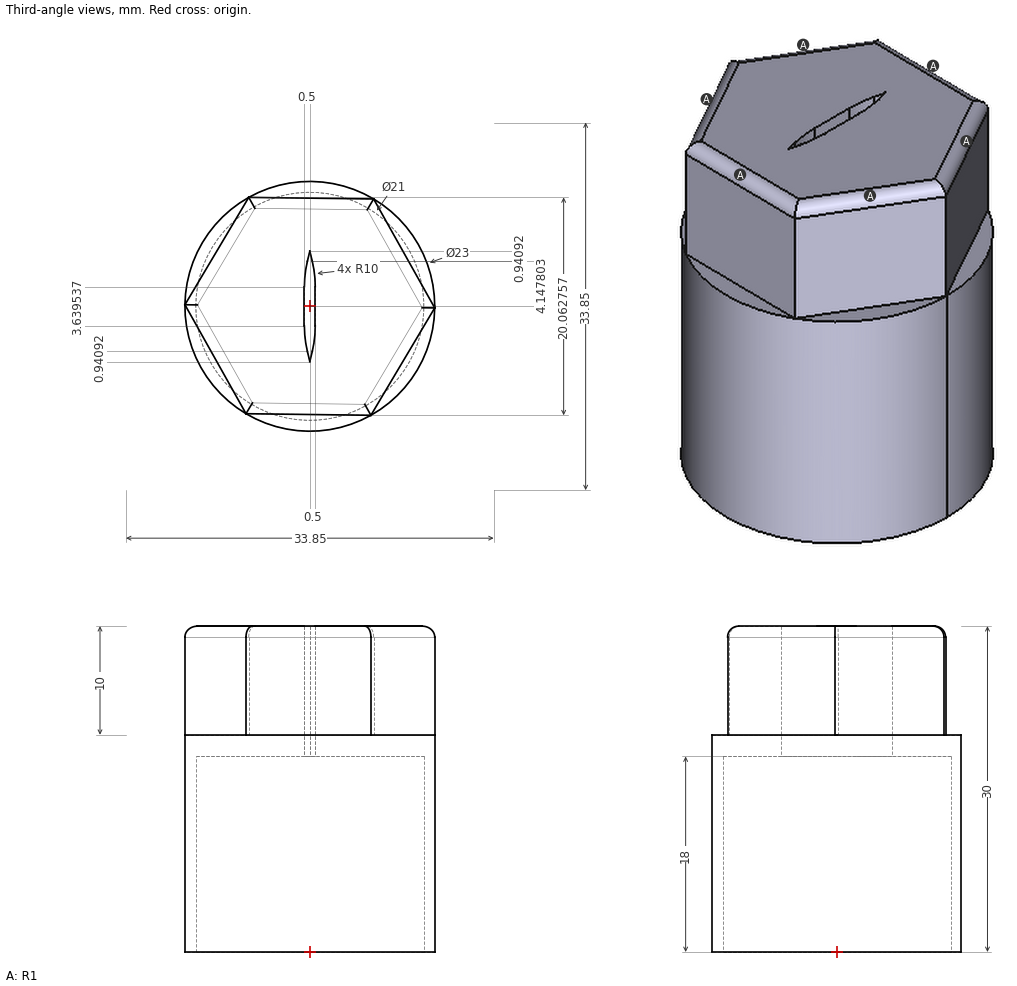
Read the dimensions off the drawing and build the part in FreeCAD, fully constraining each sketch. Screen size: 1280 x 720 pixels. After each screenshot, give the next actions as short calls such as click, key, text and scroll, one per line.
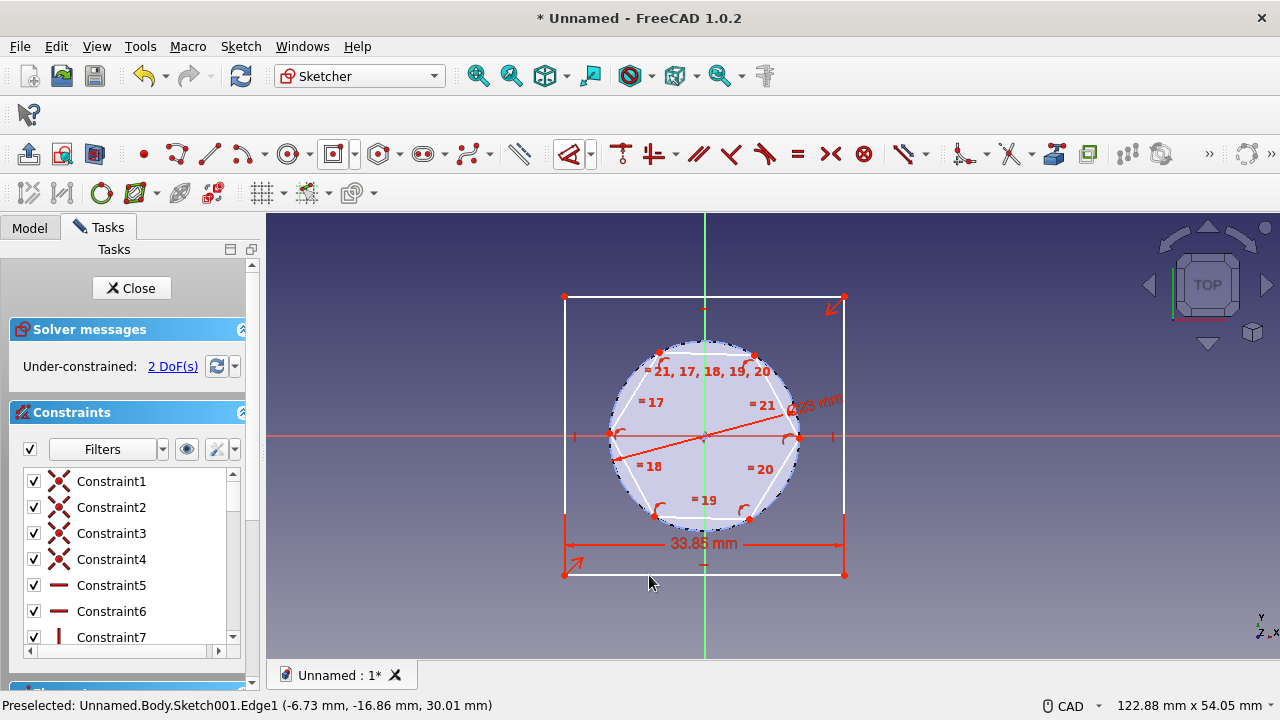
click(844, 492)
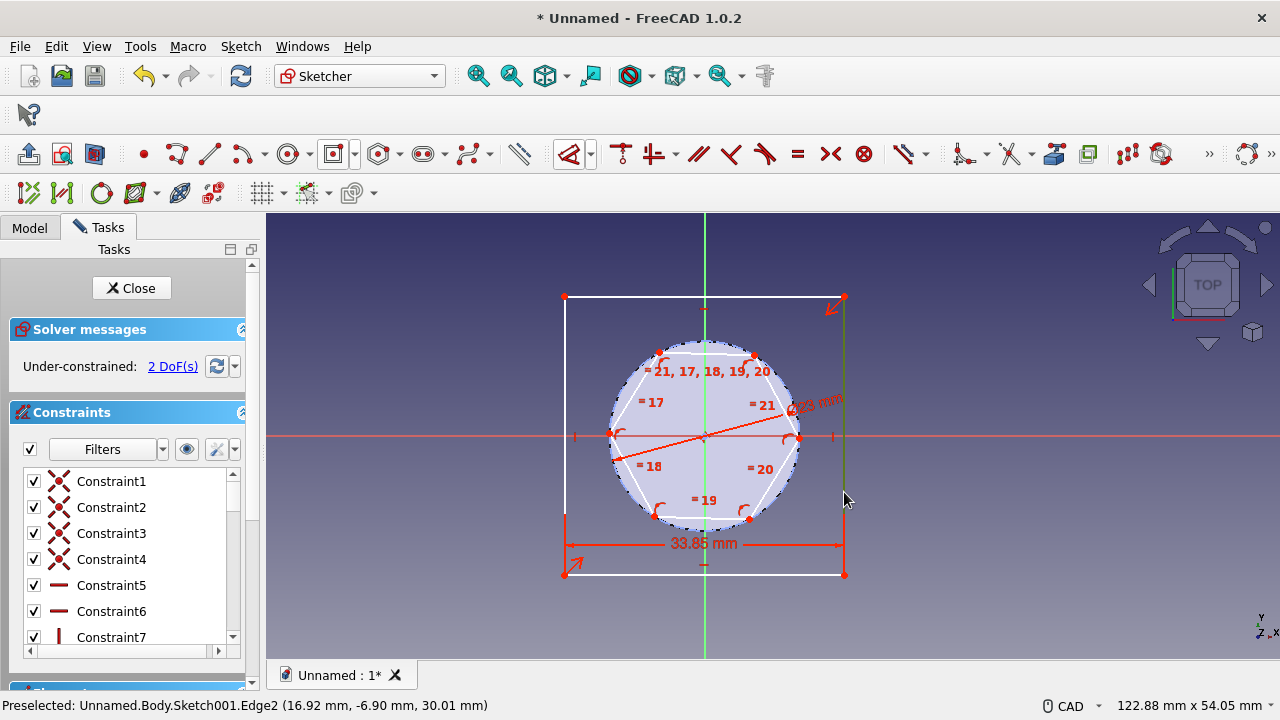
key(i)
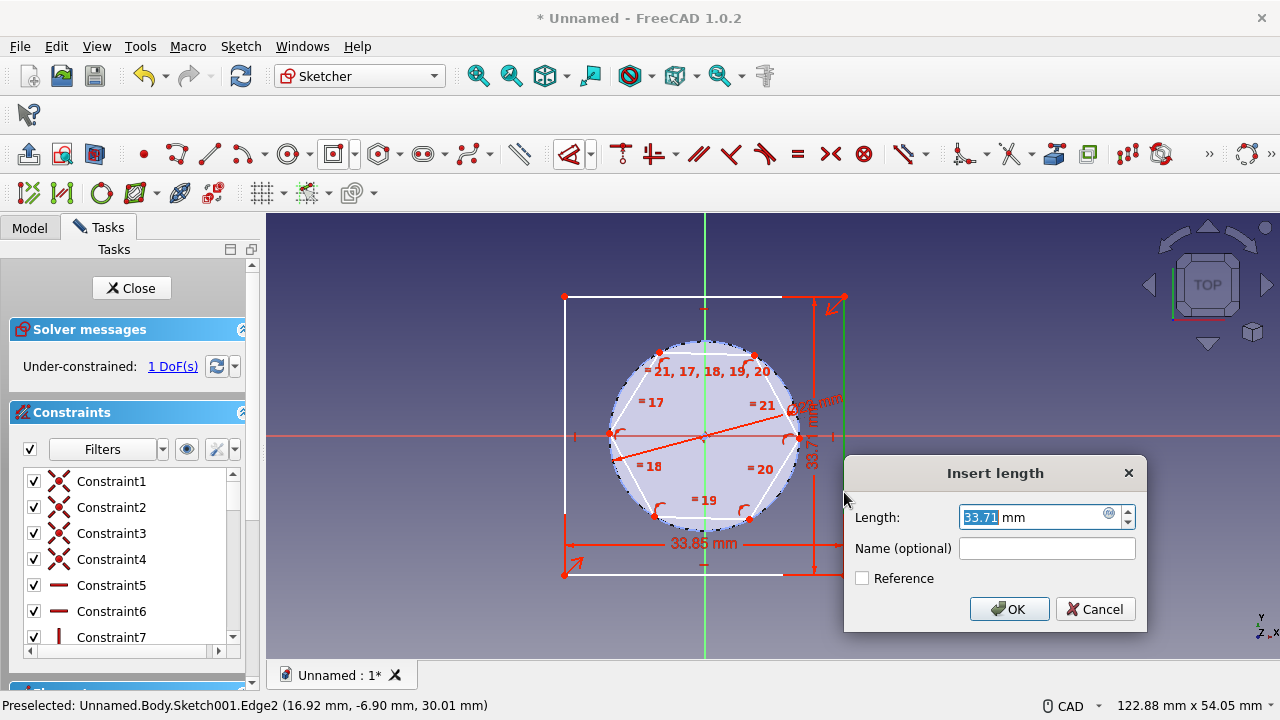
text(33.85)
key(Return)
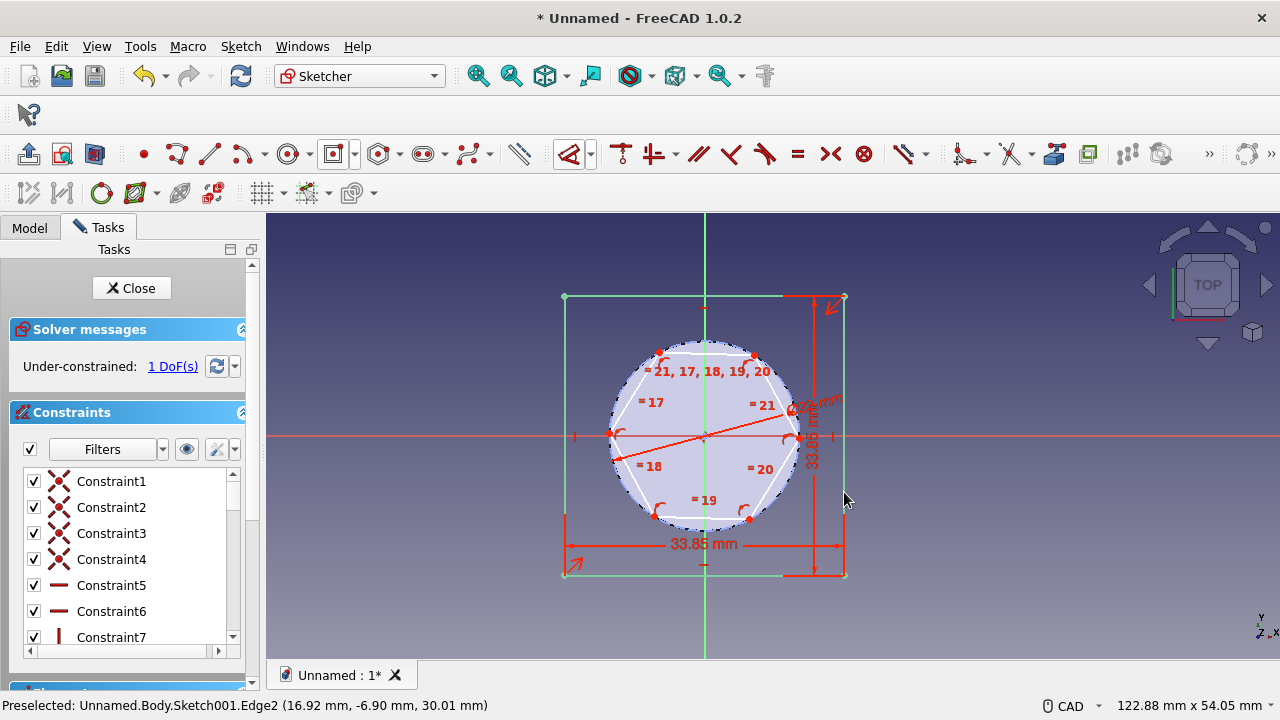
click(750, 520)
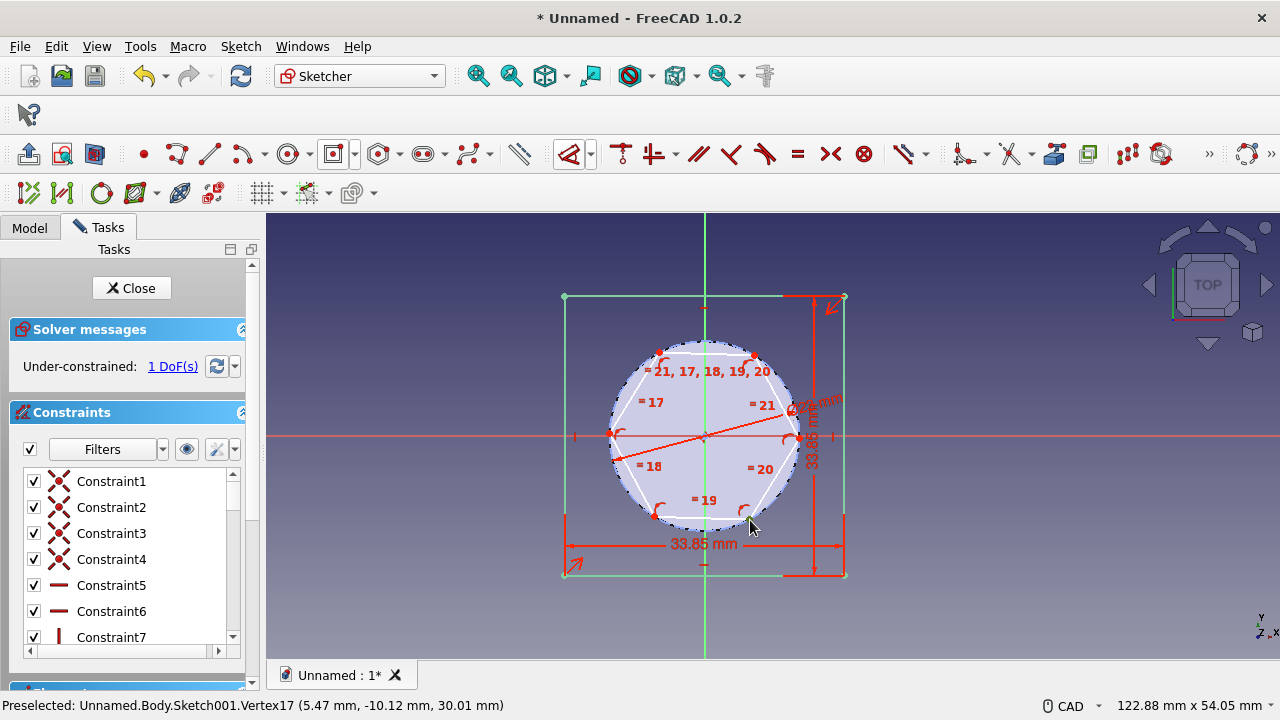
click(659, 353)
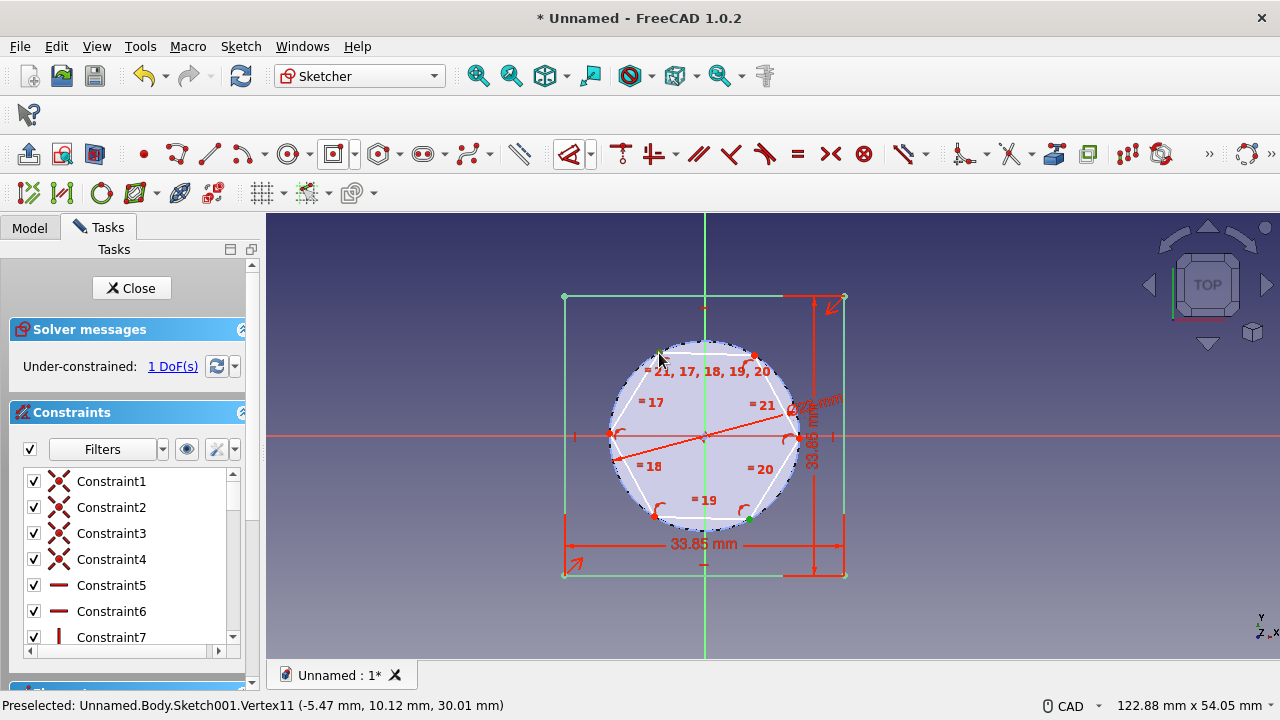
key(i)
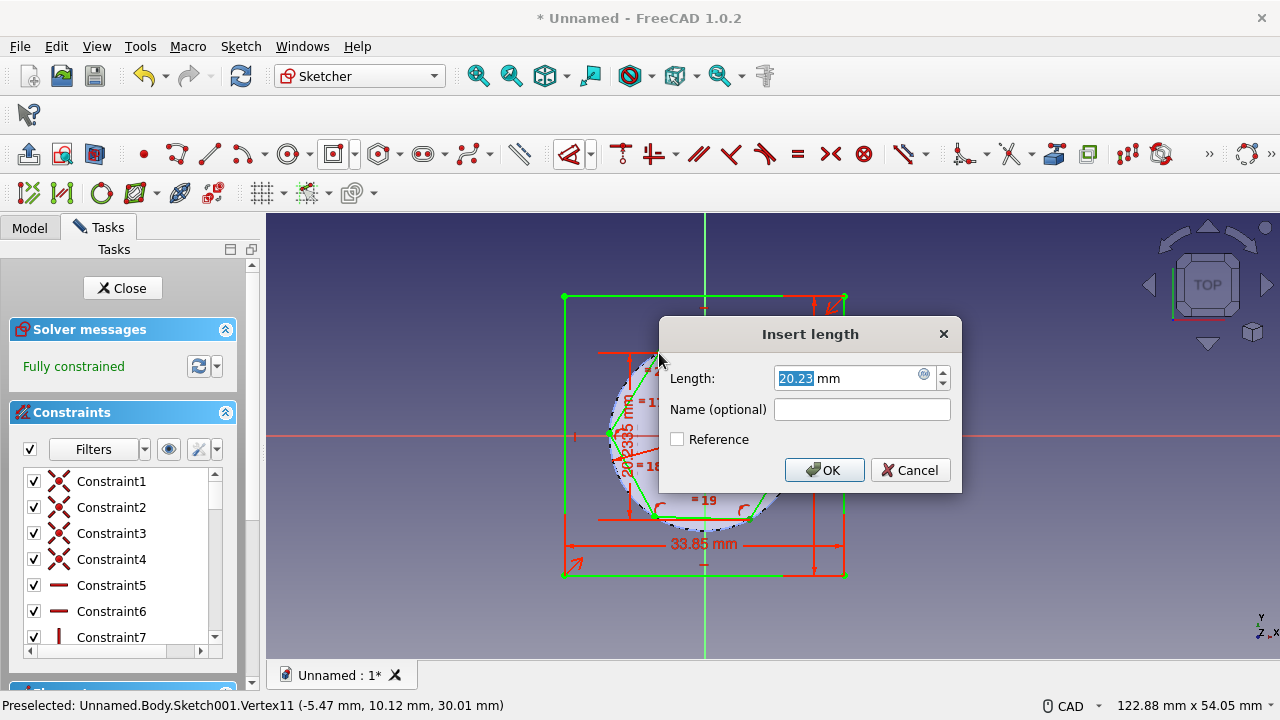
text(20.062757)
key(Return)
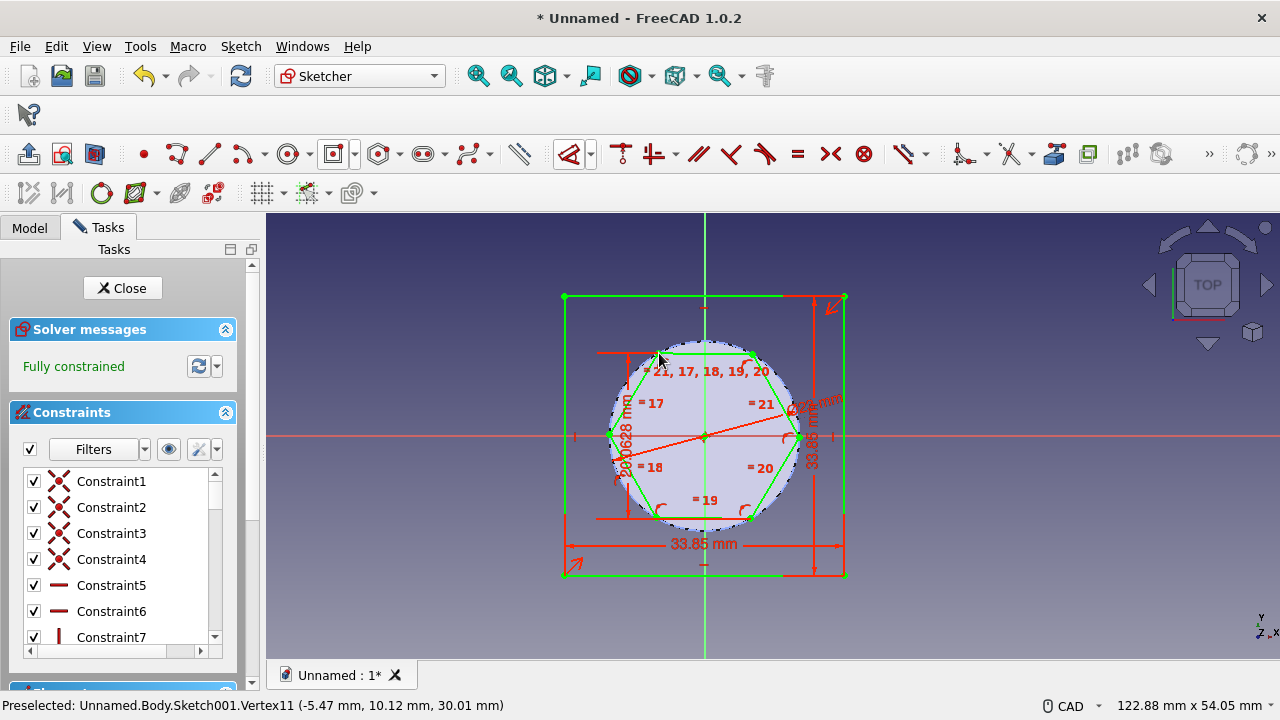
click(123, 288)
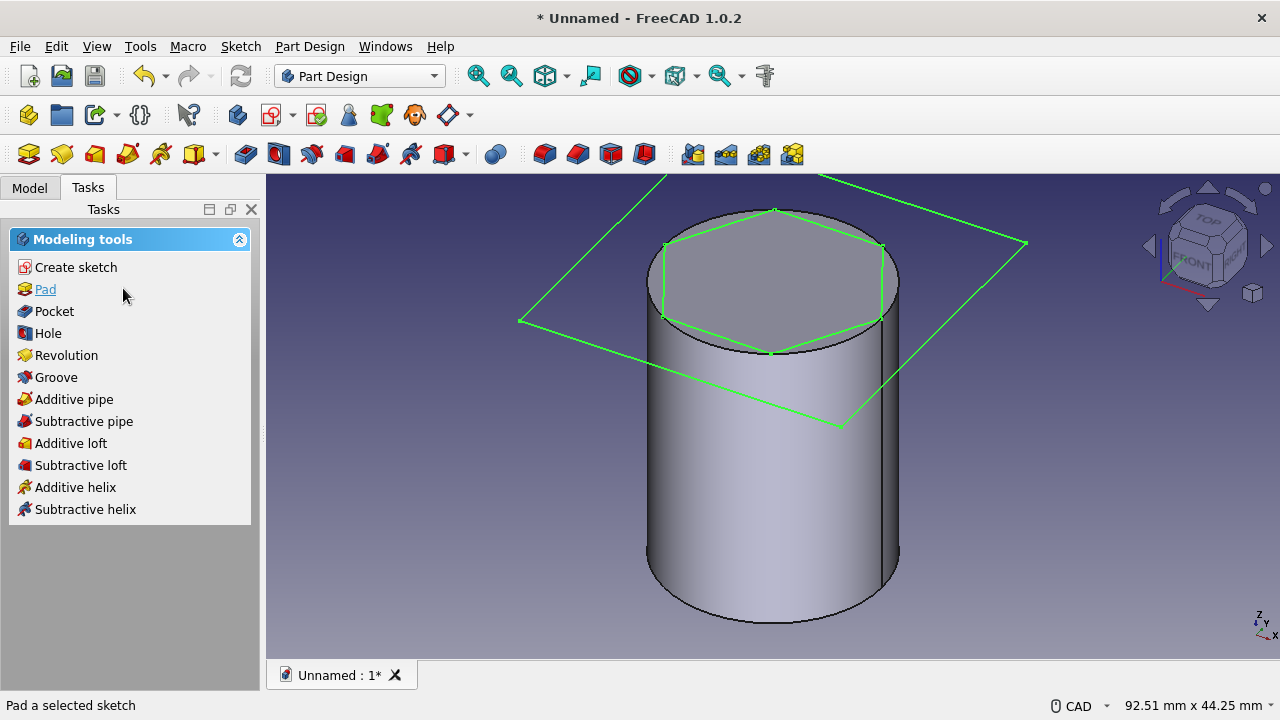
click(246, 154)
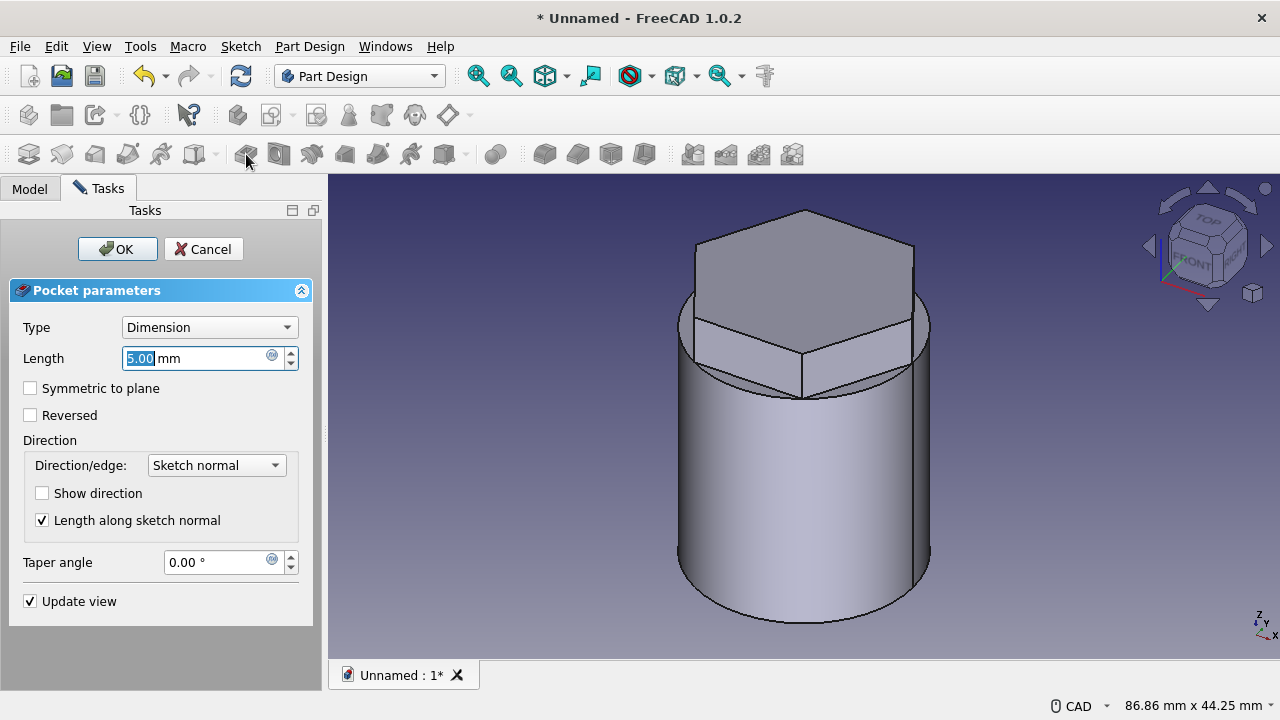
text(10)
key(Tab)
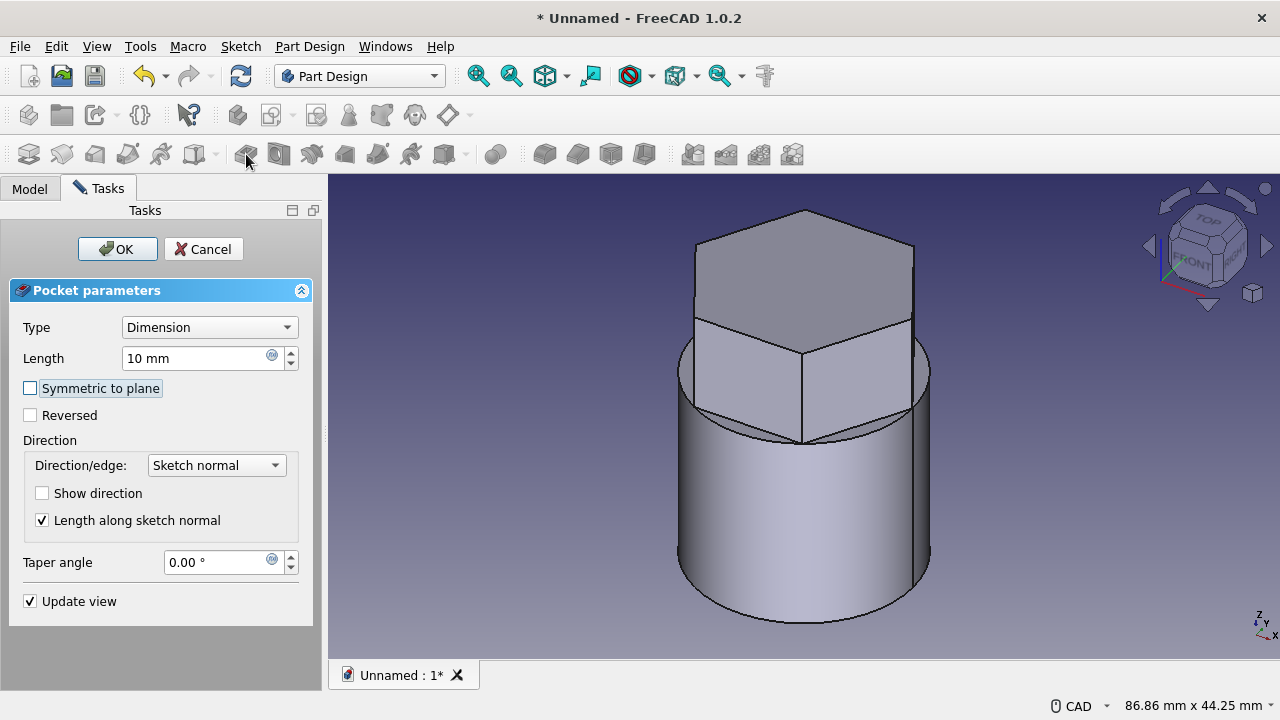
click(118, 249)